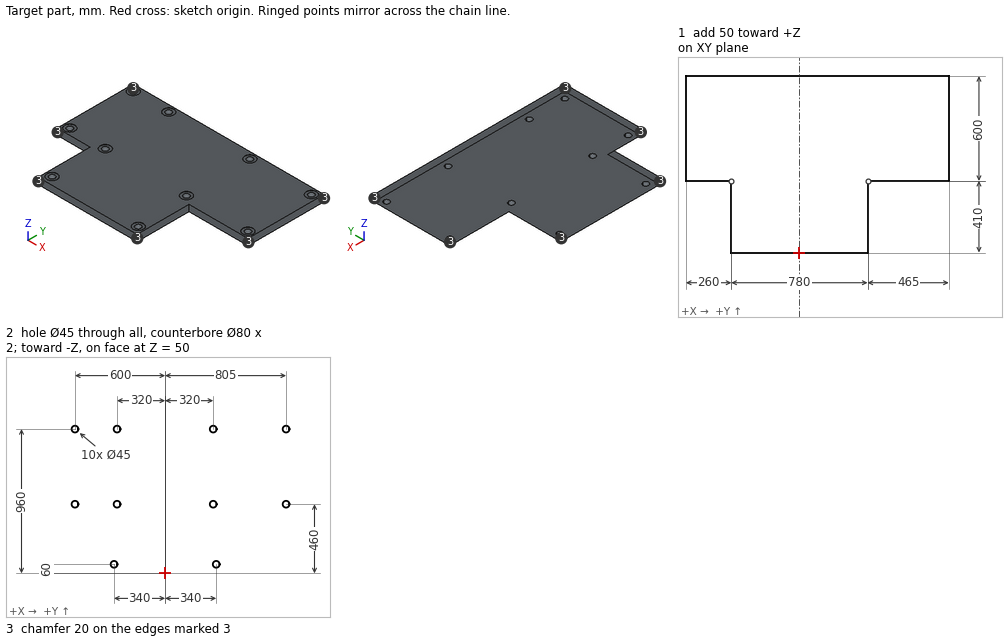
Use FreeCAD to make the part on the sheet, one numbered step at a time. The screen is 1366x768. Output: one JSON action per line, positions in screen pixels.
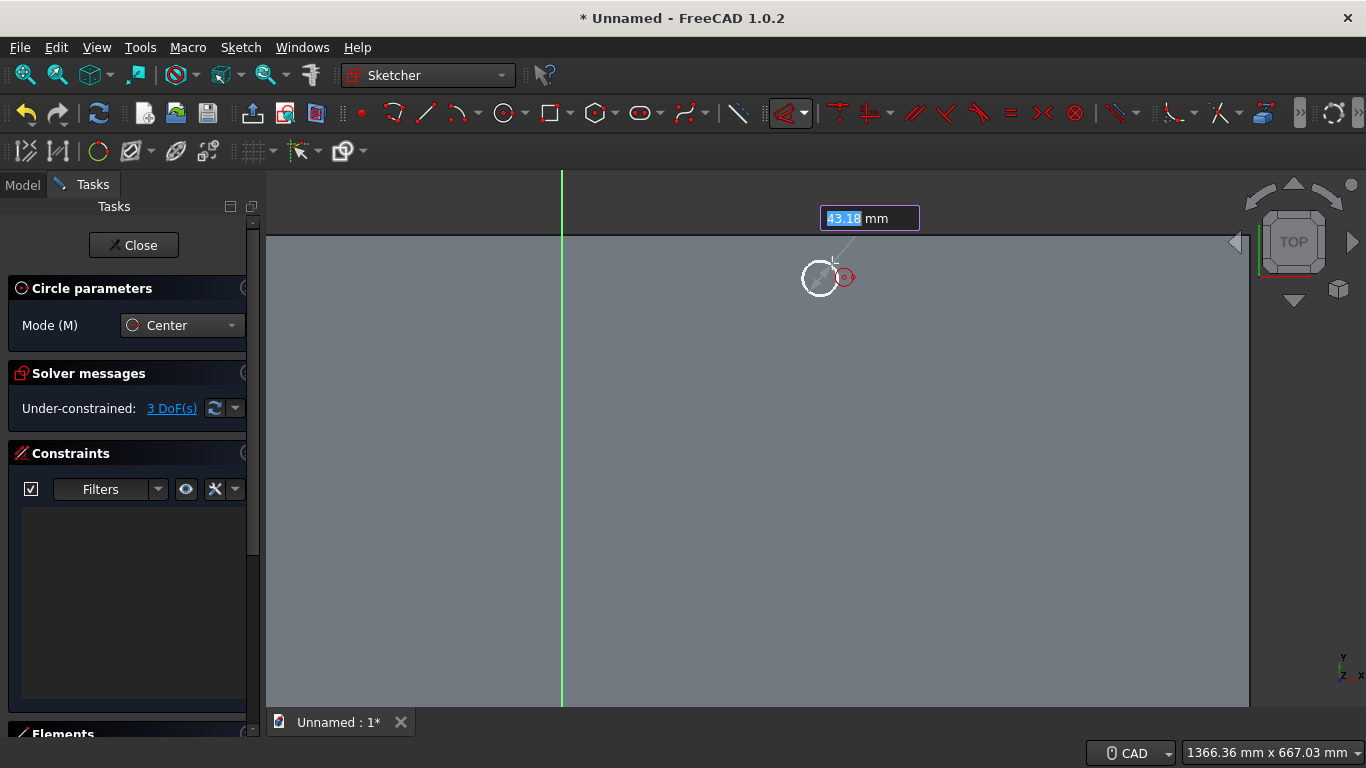
{"action": "left_click", "coordinate": [832, 263]}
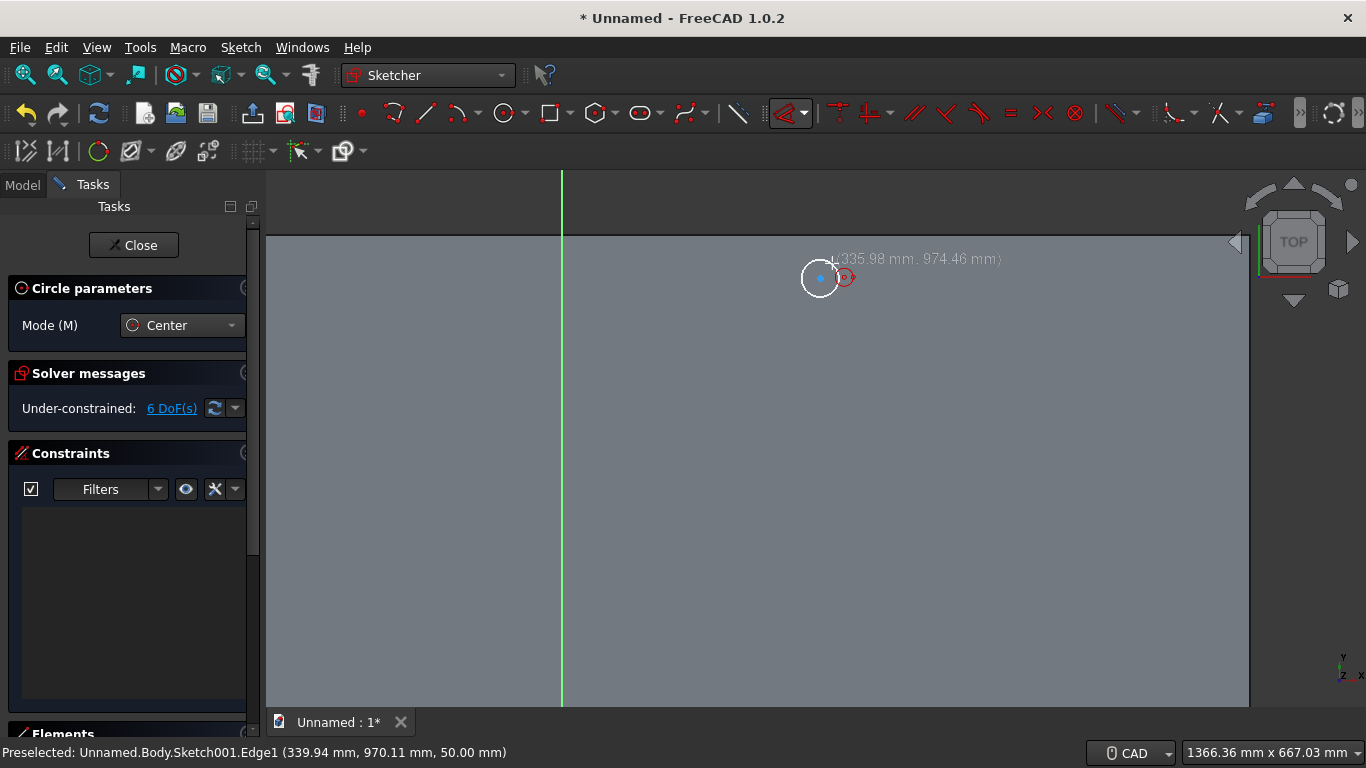
{"action": "scroll", "coordinate": [832, 263], "scroll_direction": "down", "scroll_amount": 4}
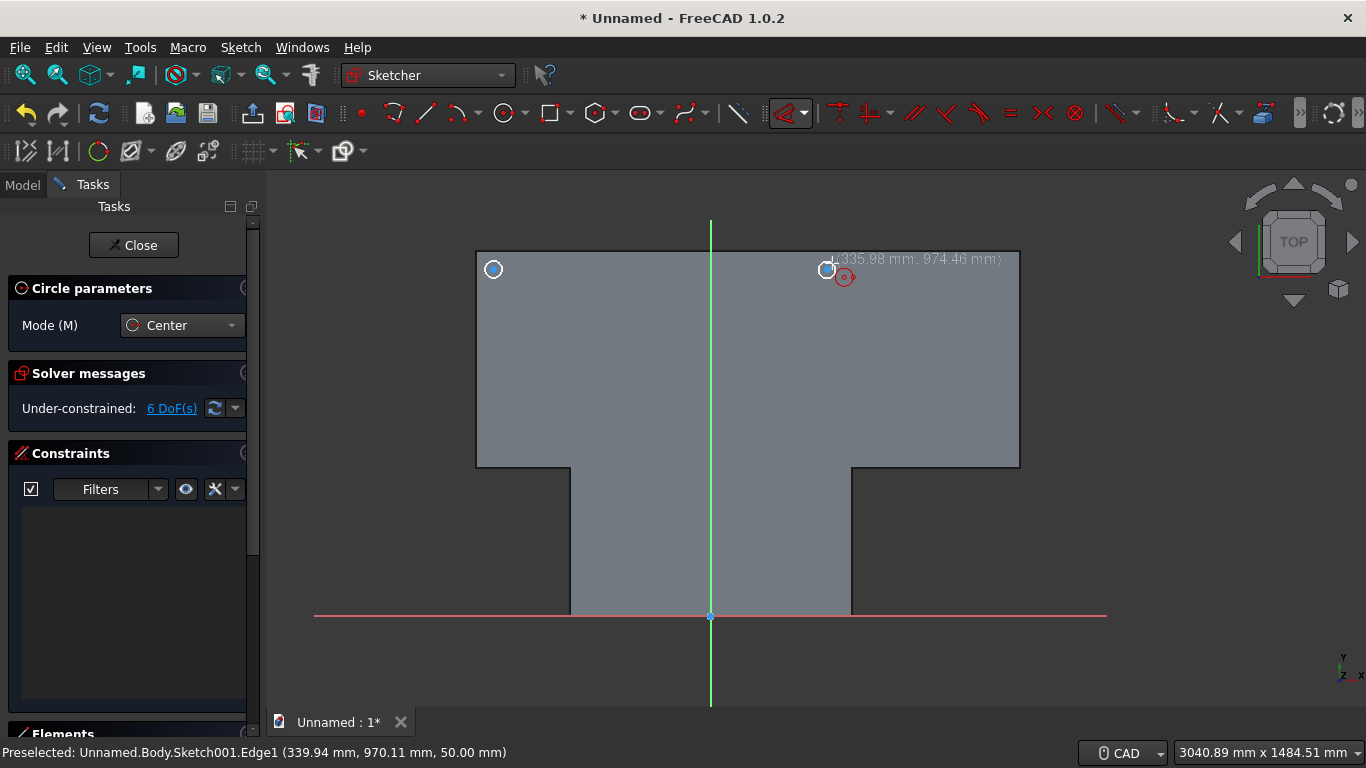
{"action": "scroll", "coordinate": [1002, 269], "scroll_direction": "up", "scroll_amount": 6}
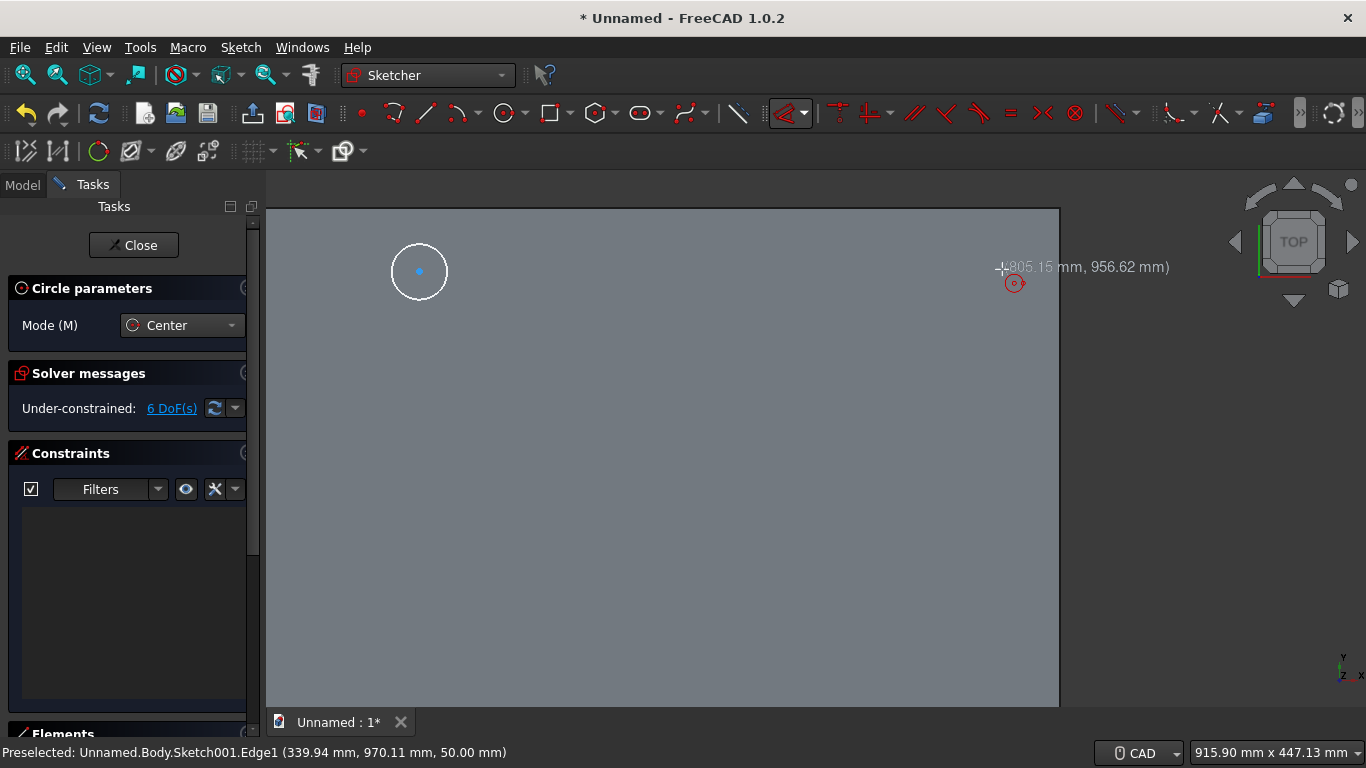
{"action": "scroll", "coordinate": [1002, 269], "scroll_direction": "down", "scroll_amount": 6}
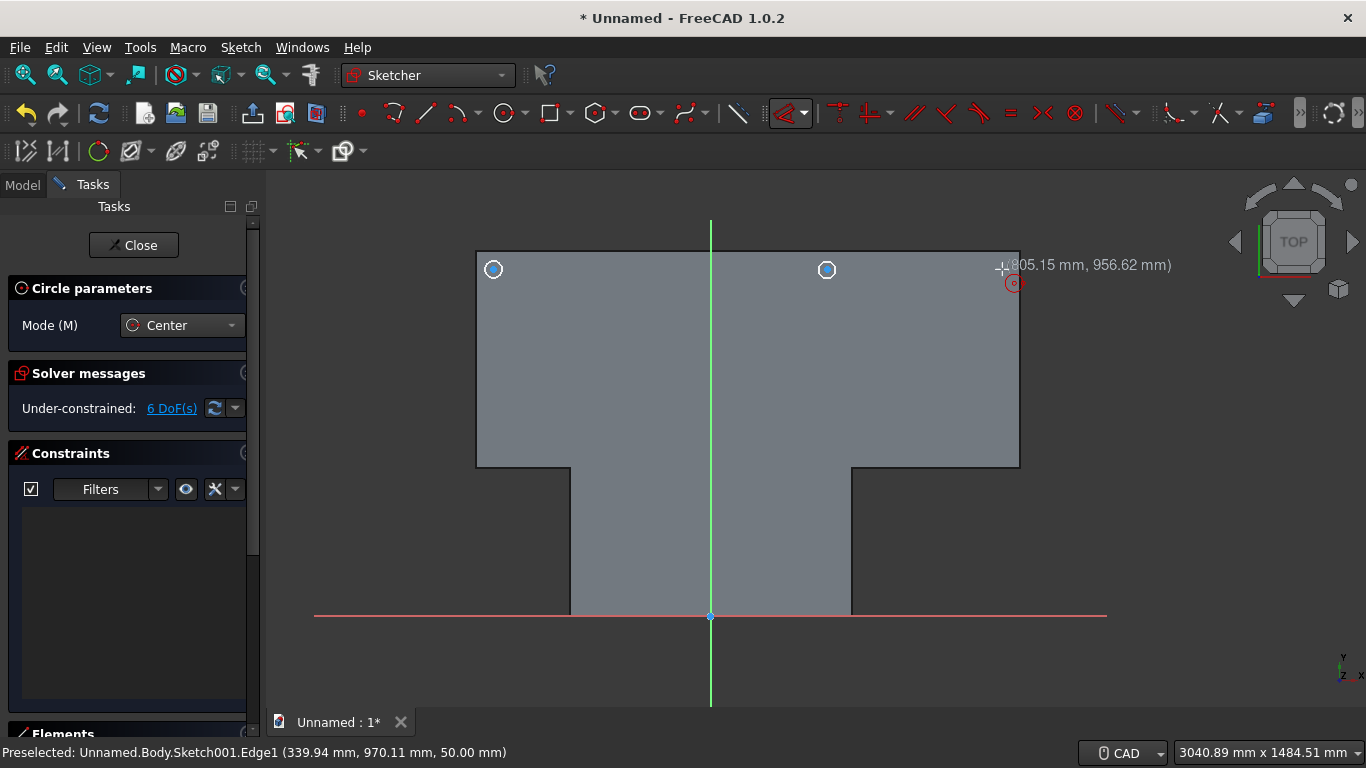
{"action": "left_click", "coordinate": [1002, 269]}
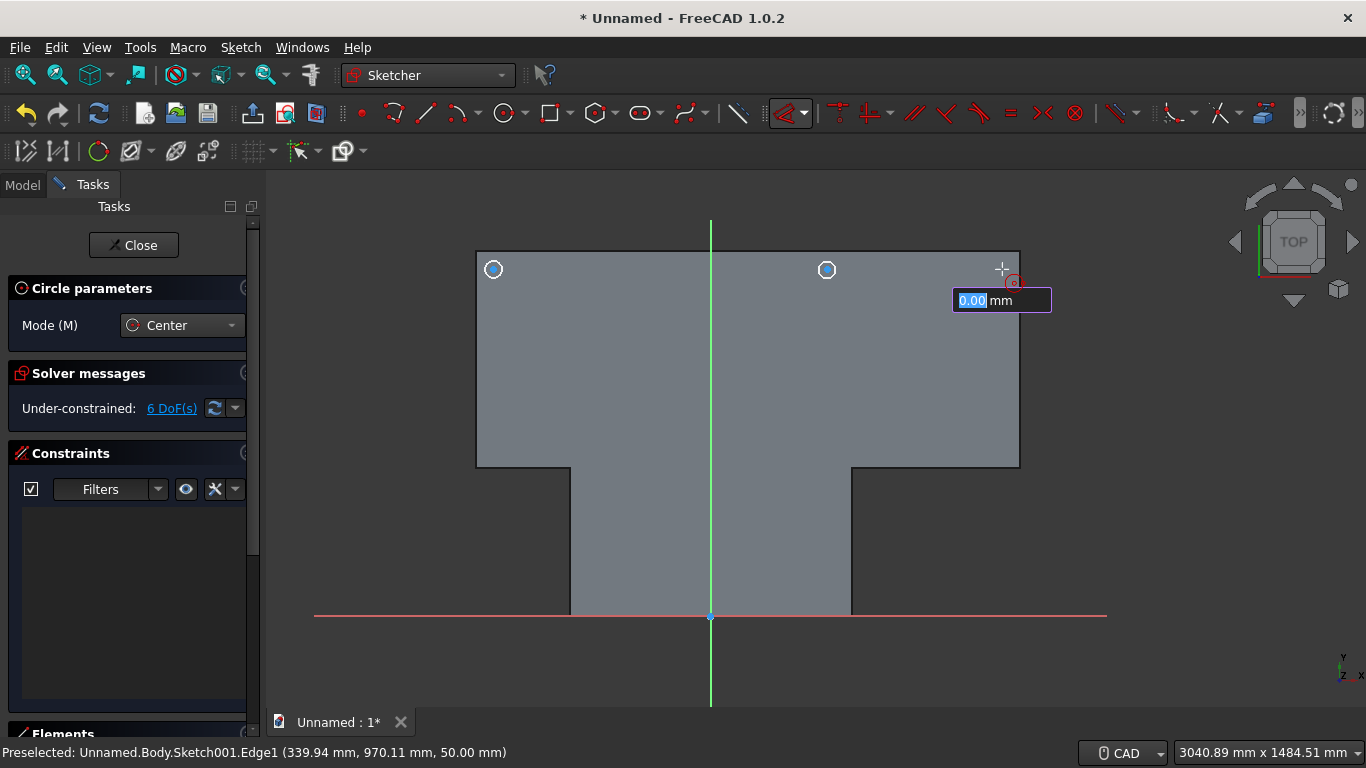
{"action": "scroll", "coordinate": [1008, 263], "scroll_direction": "up", "scroll_amount": 4}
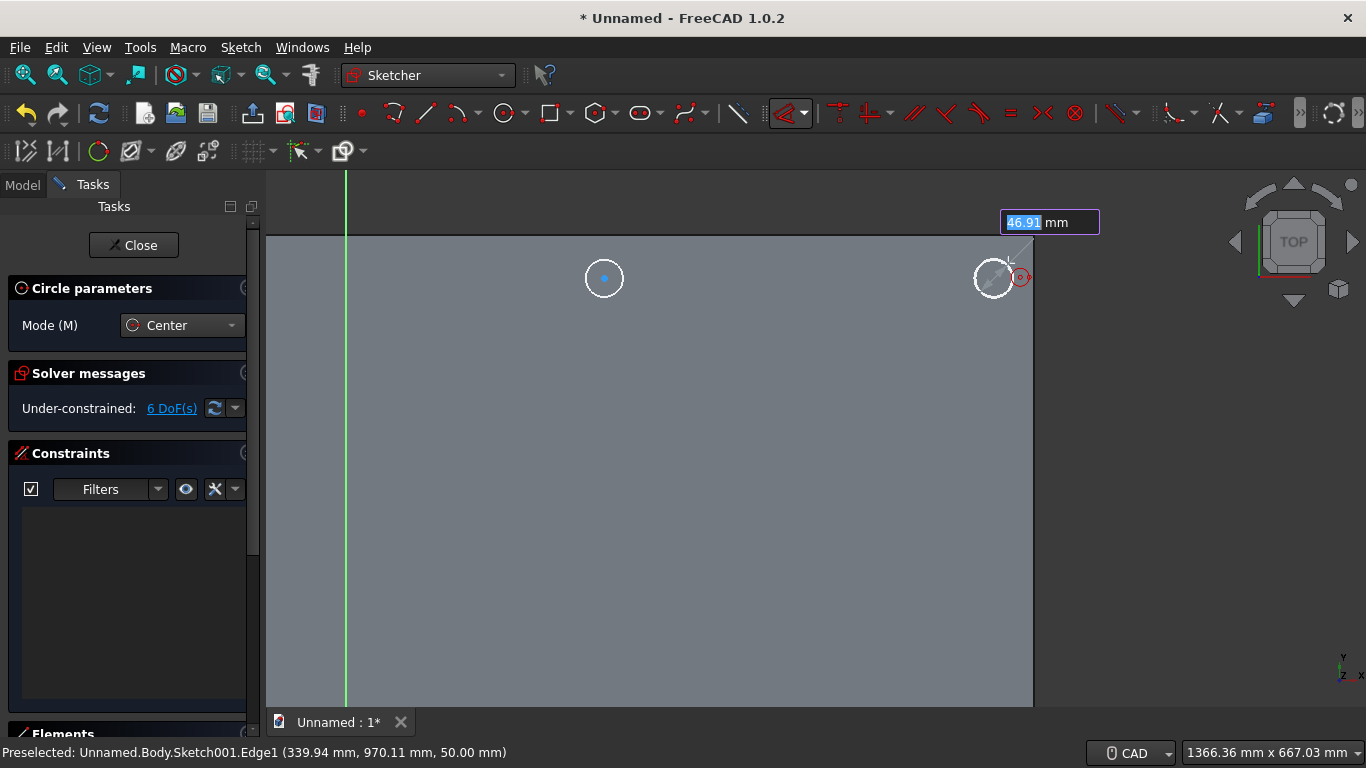
{"action": "left_click", "coordinate": [1007, 263]}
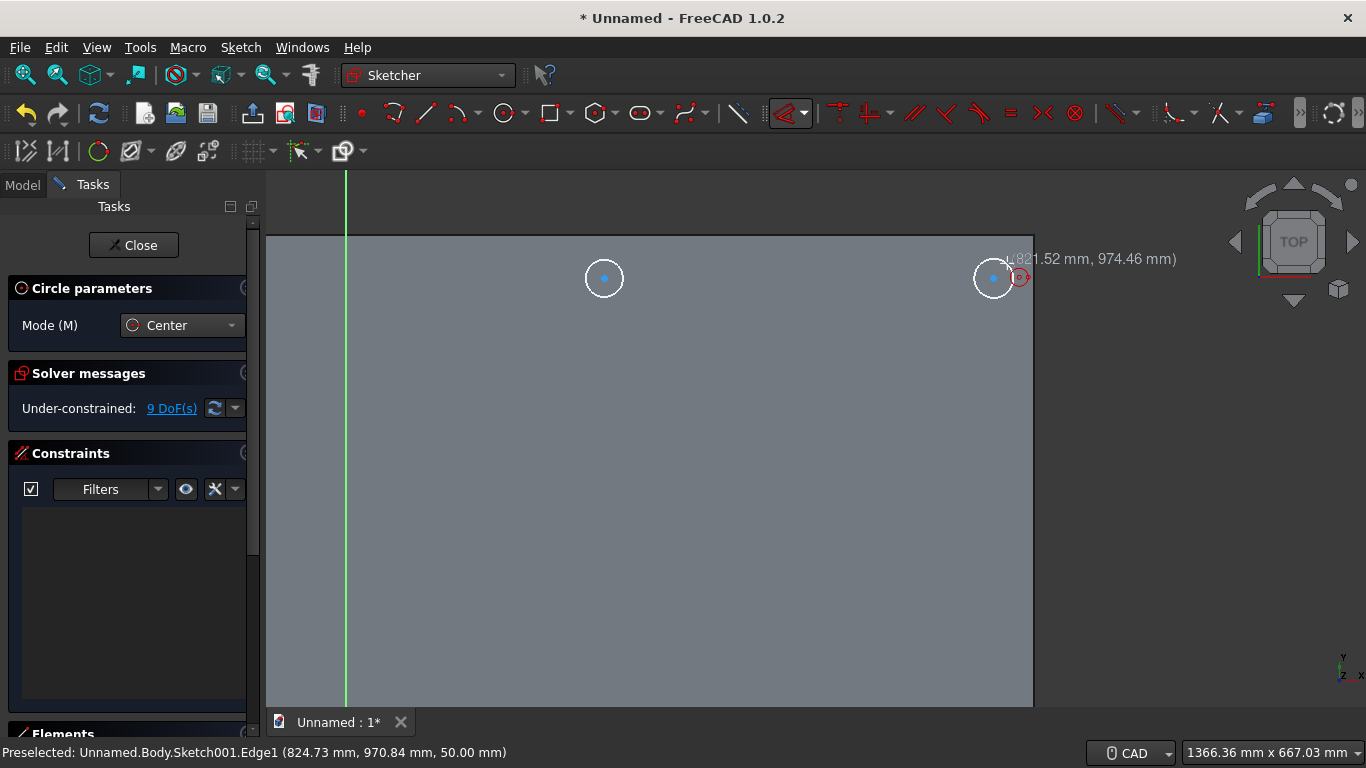
{"action": "scroll", "coordinate": [1008, 263], "scroll_direction": "down", "scroll_amount": 4}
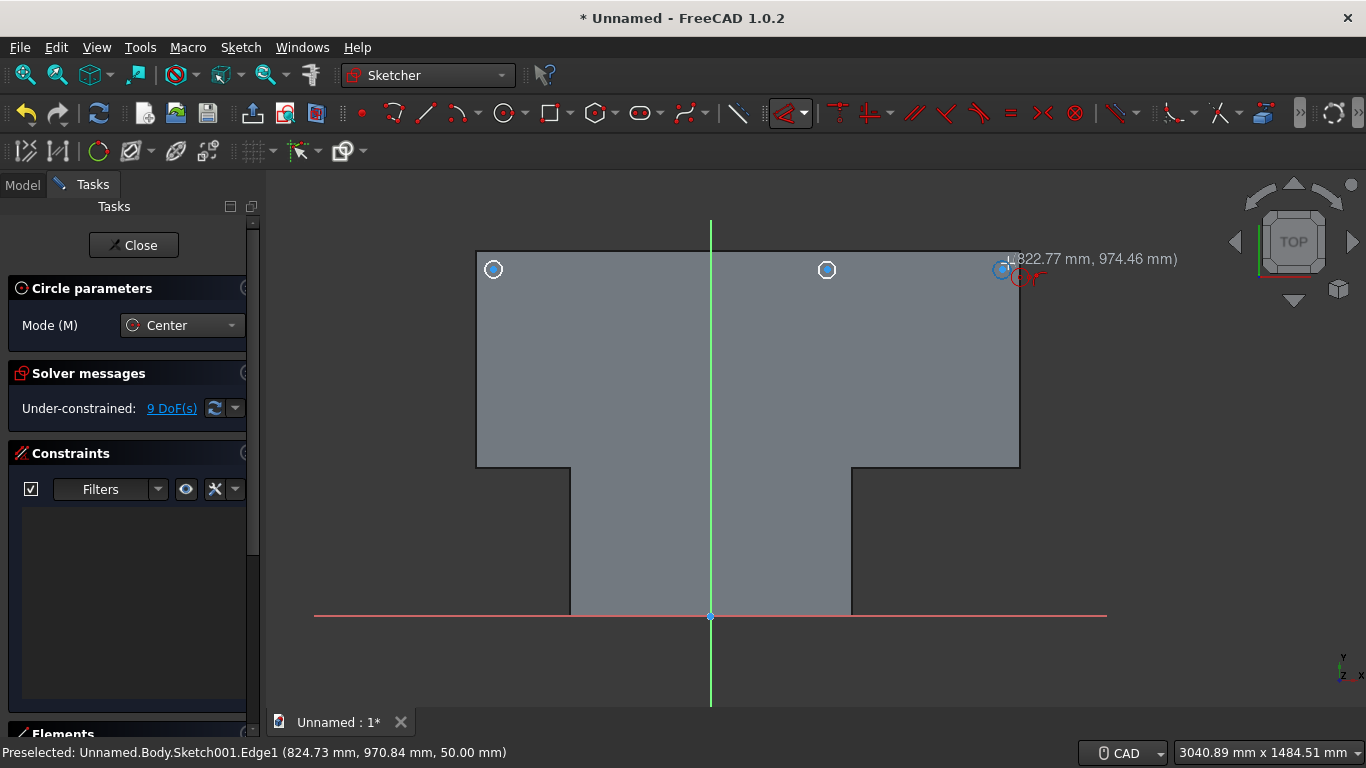
{"action": "scroll", "coordinate": [588, 594], "scroll_direction": "up", "scroll_amount": 6}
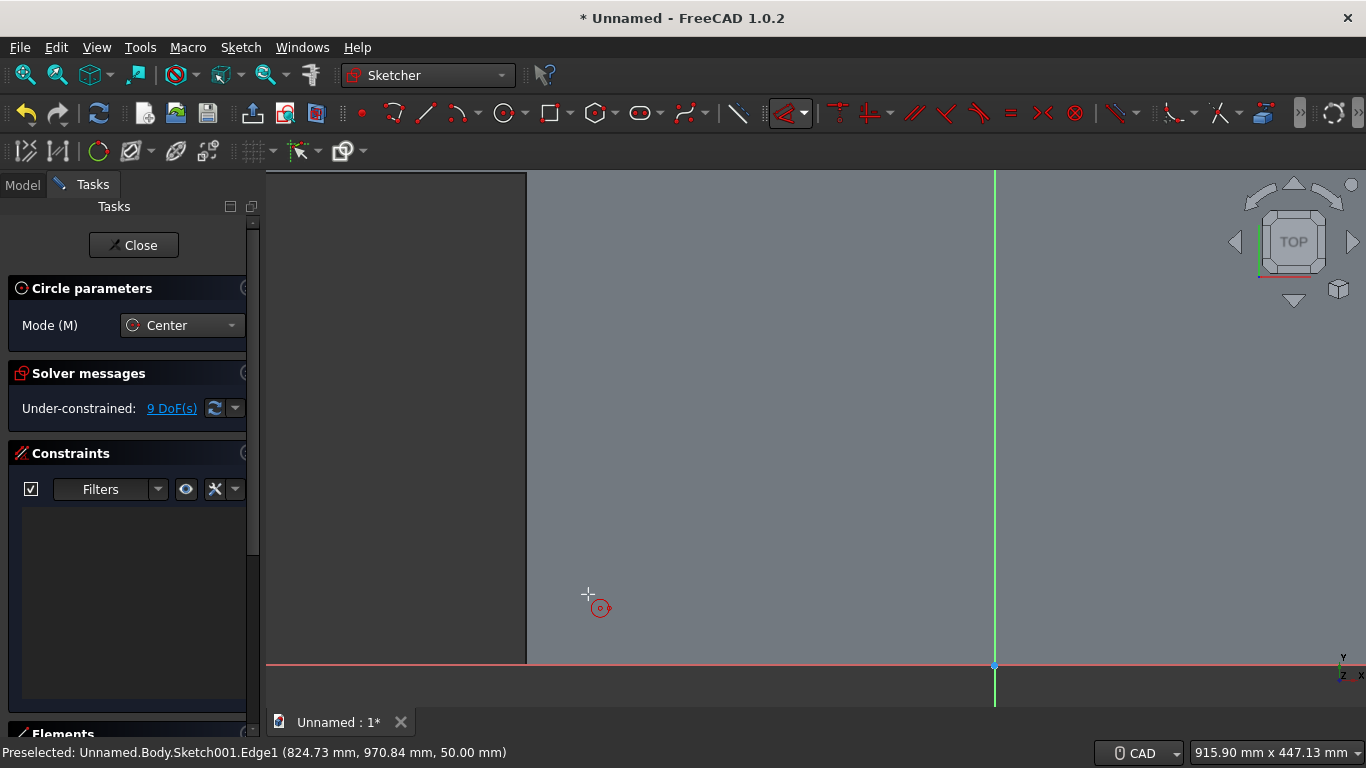
{"action": "scroll", "coordinate": [588, 595], "scroll_direction": "down", "scroll_amount": 6}